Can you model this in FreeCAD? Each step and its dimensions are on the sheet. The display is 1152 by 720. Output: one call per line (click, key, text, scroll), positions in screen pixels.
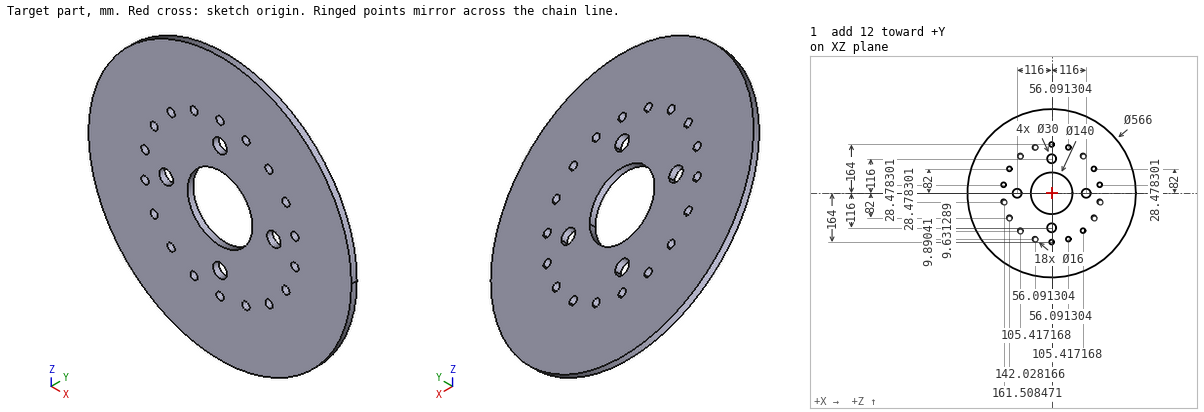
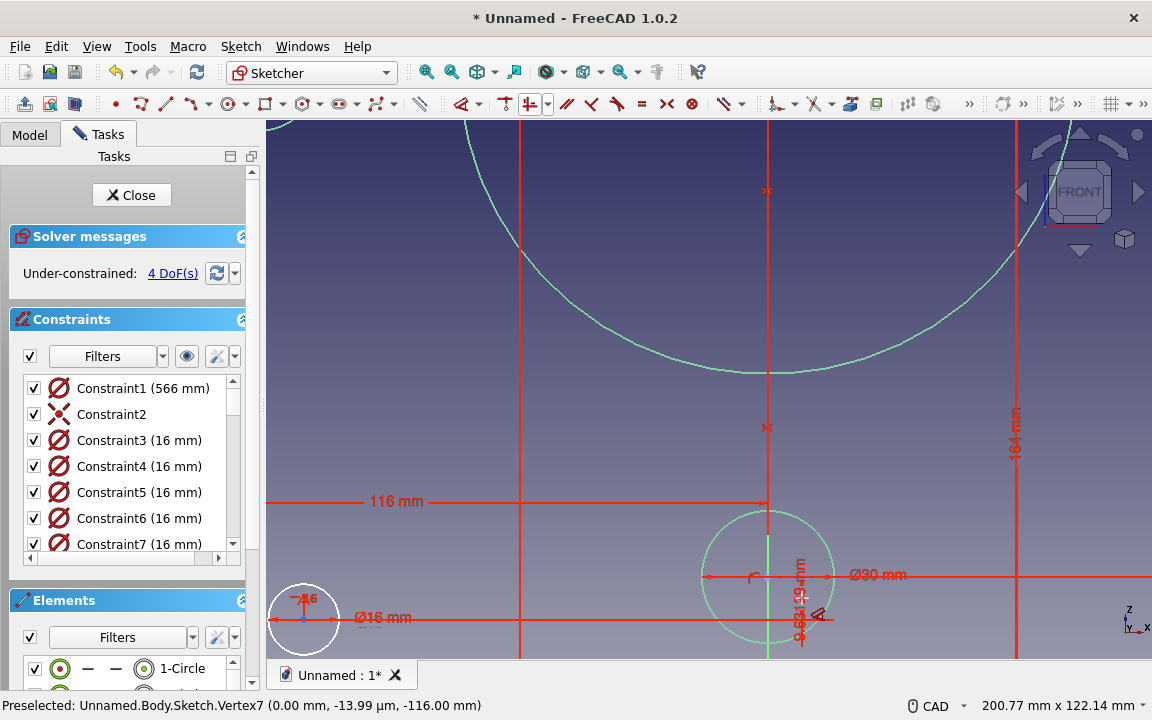
scroll(621, 440, down, 10)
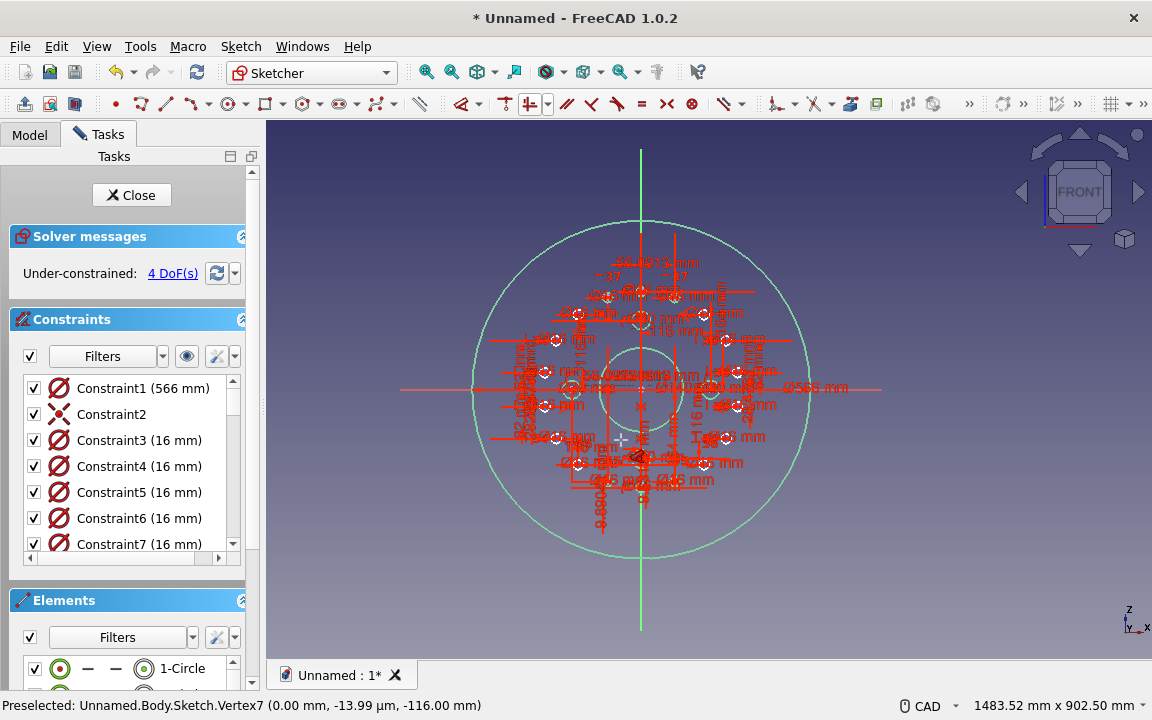
click(578, 465)
click(610, 523)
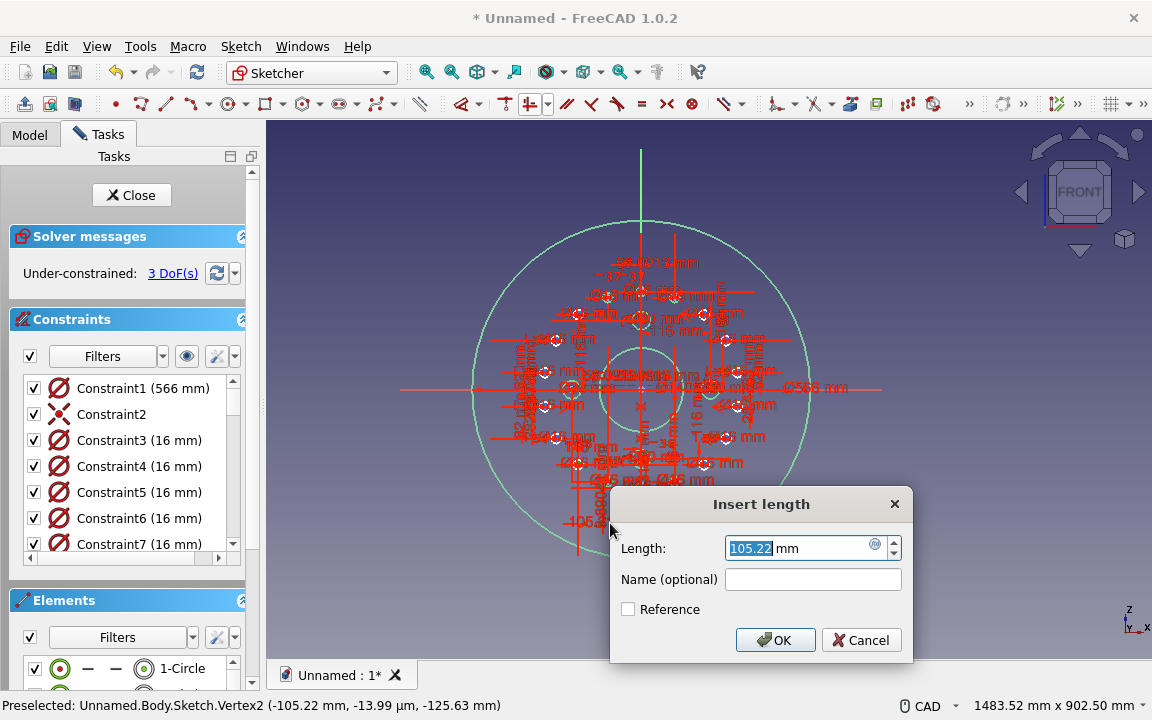
text(105.417168)
key(Return)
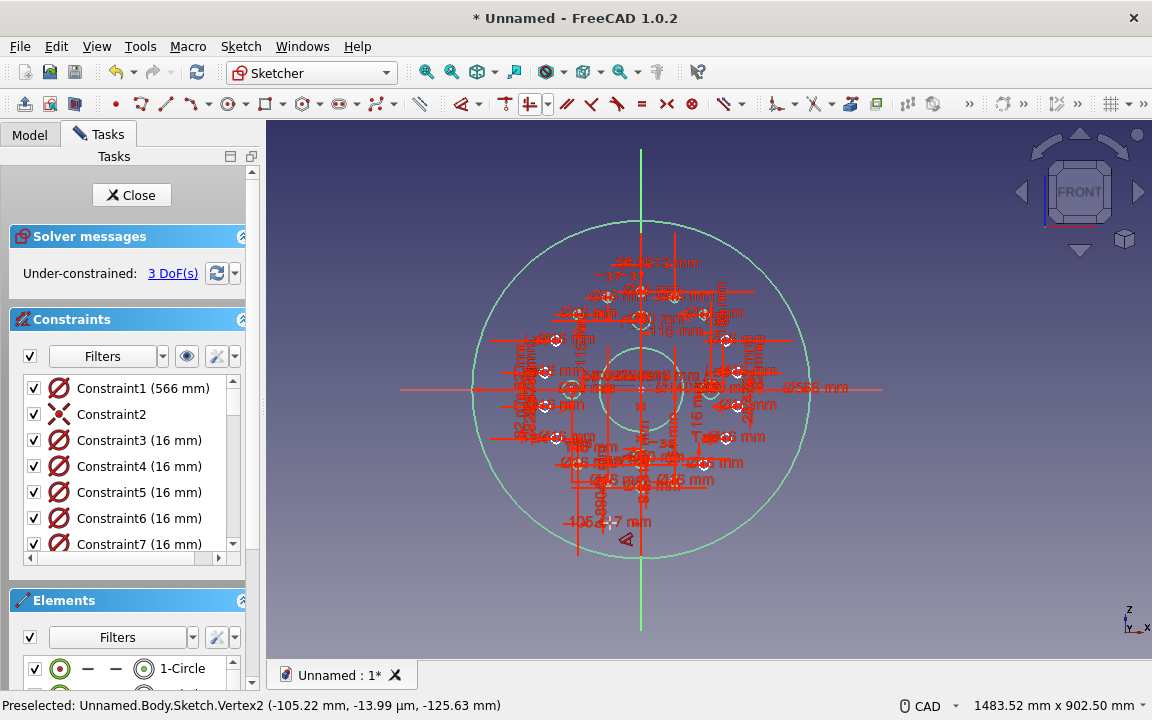
click(556, 439)
click(579, 284)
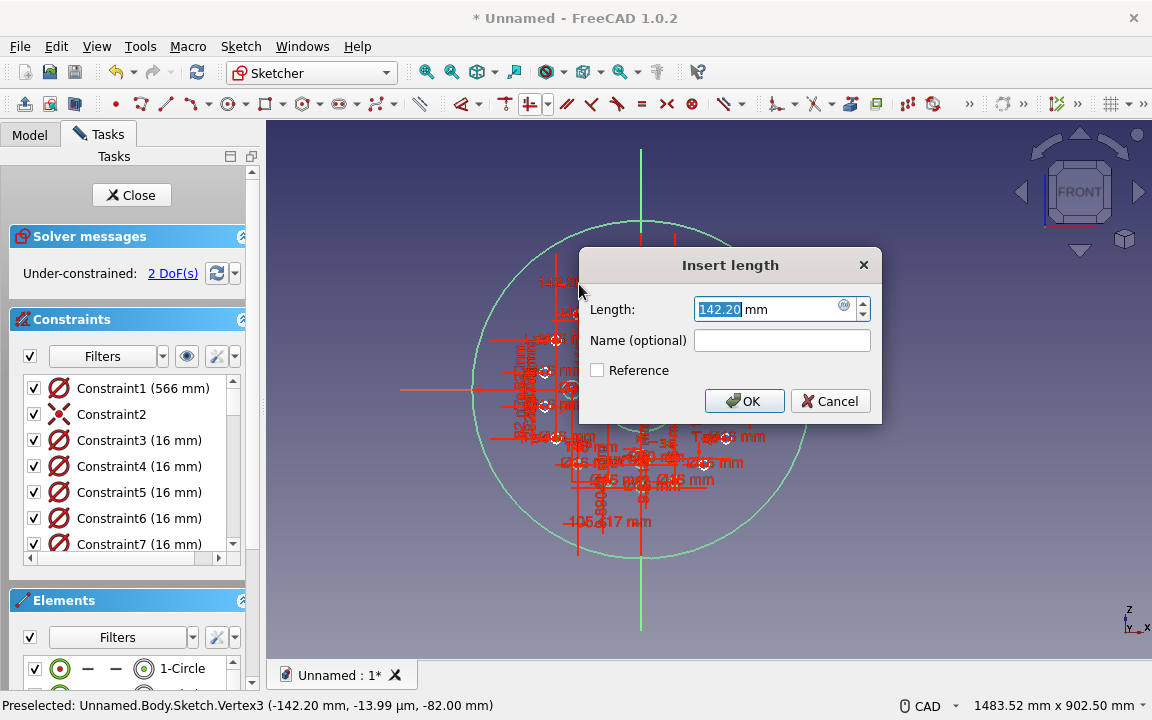
text(142.028166)
key(Return)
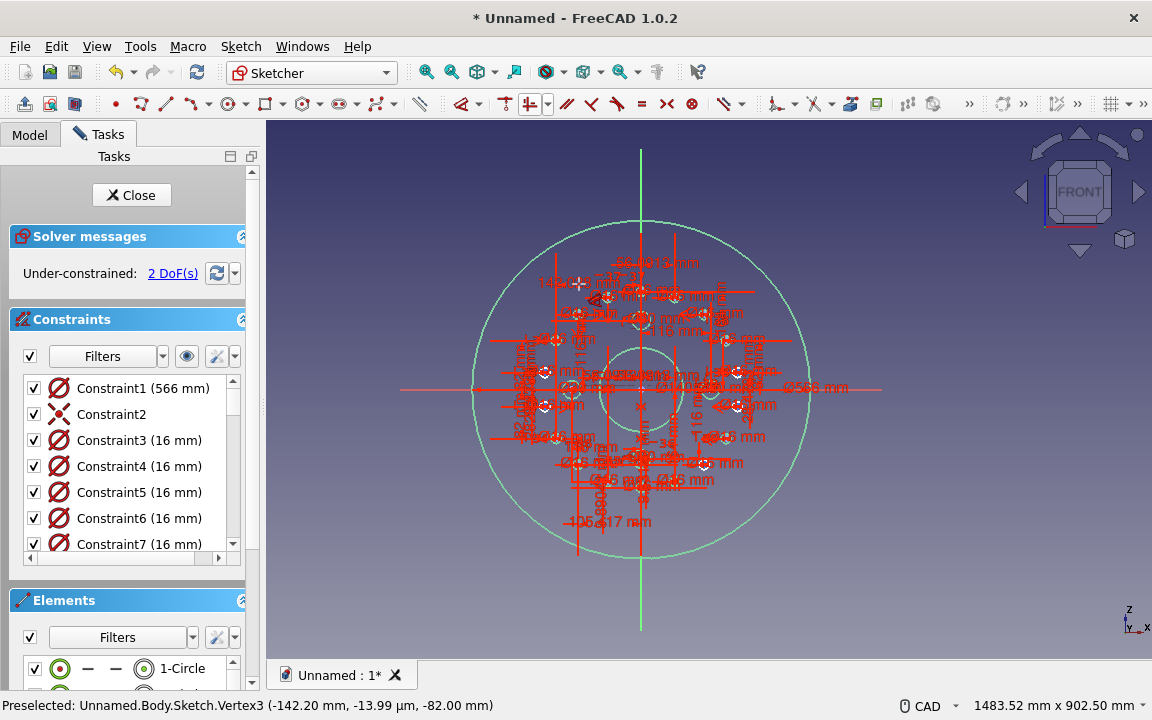
click(545, 407)
click(559, 308)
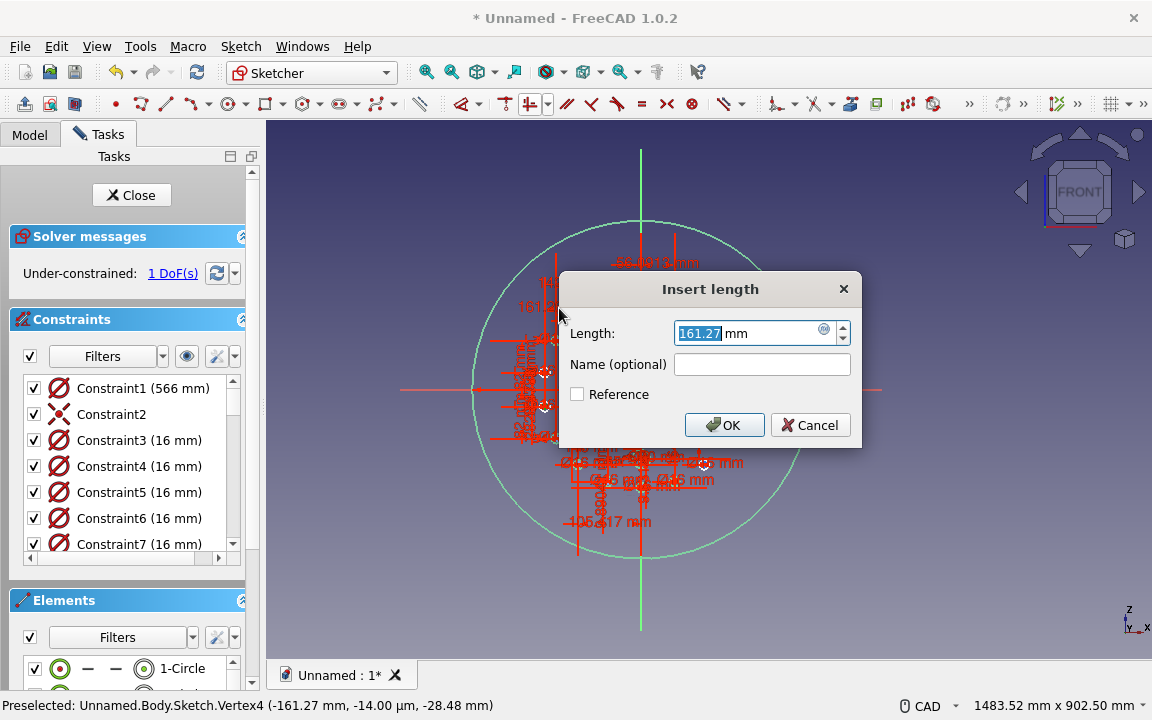
text(161.508471)
key(Return)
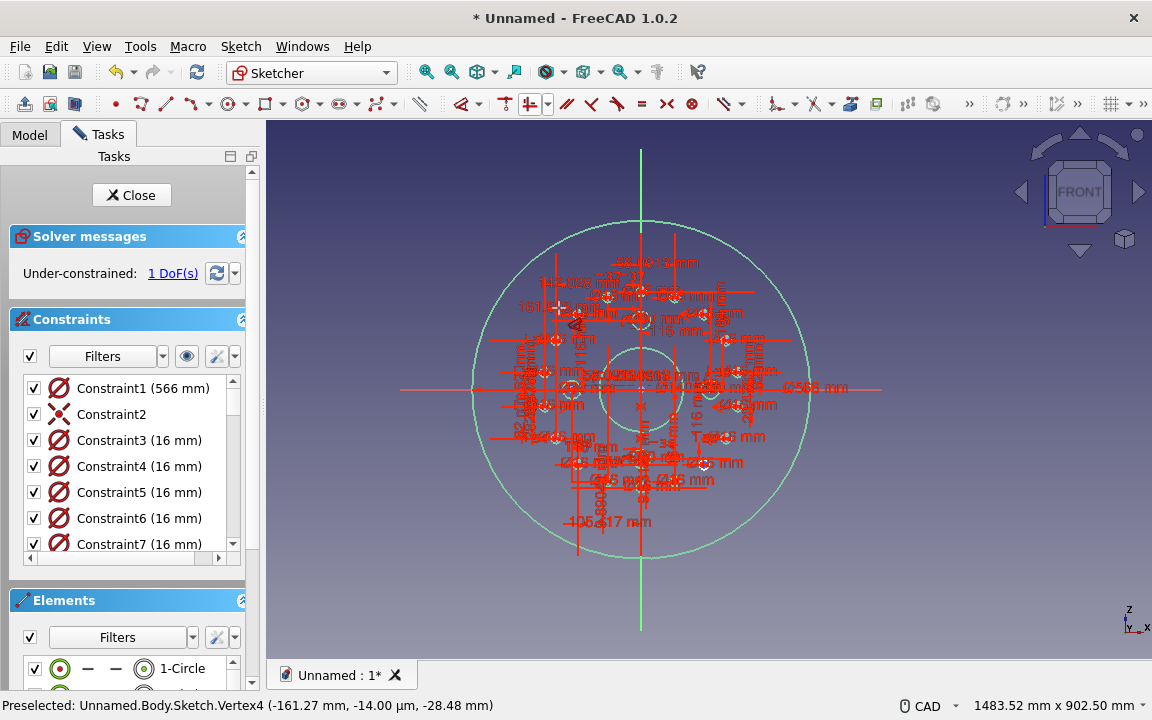
click(704, 465)
click(687, 499)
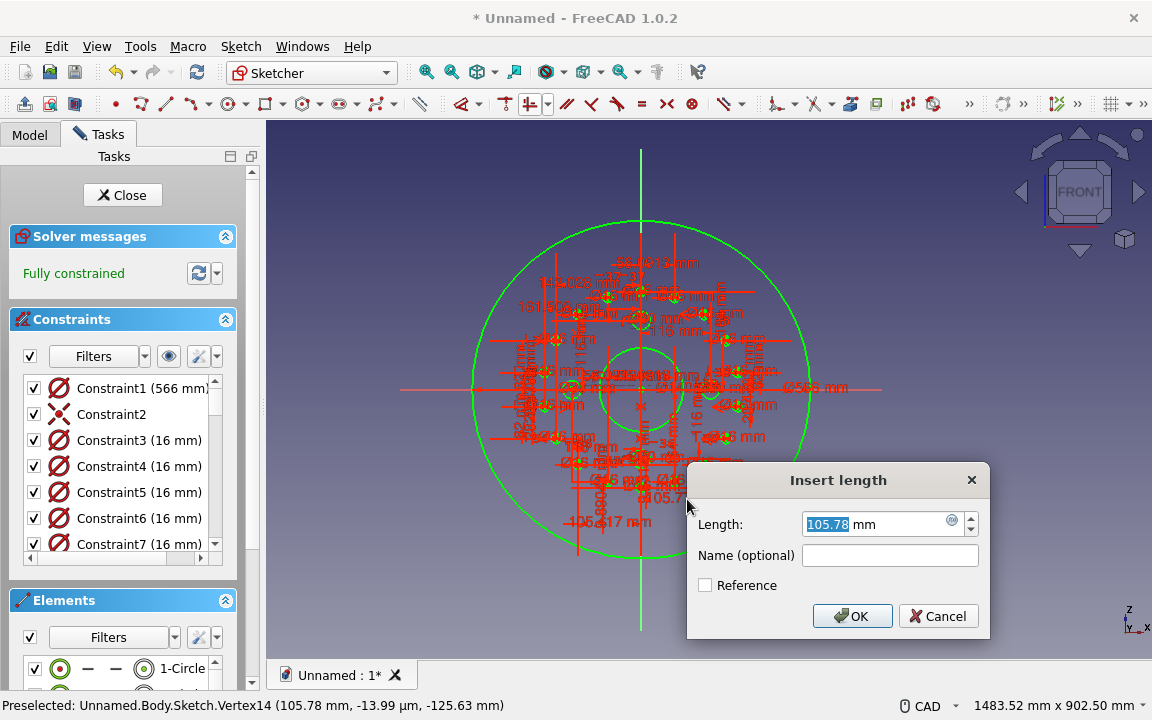
text(105.417168)
key(Return)
key(Escape)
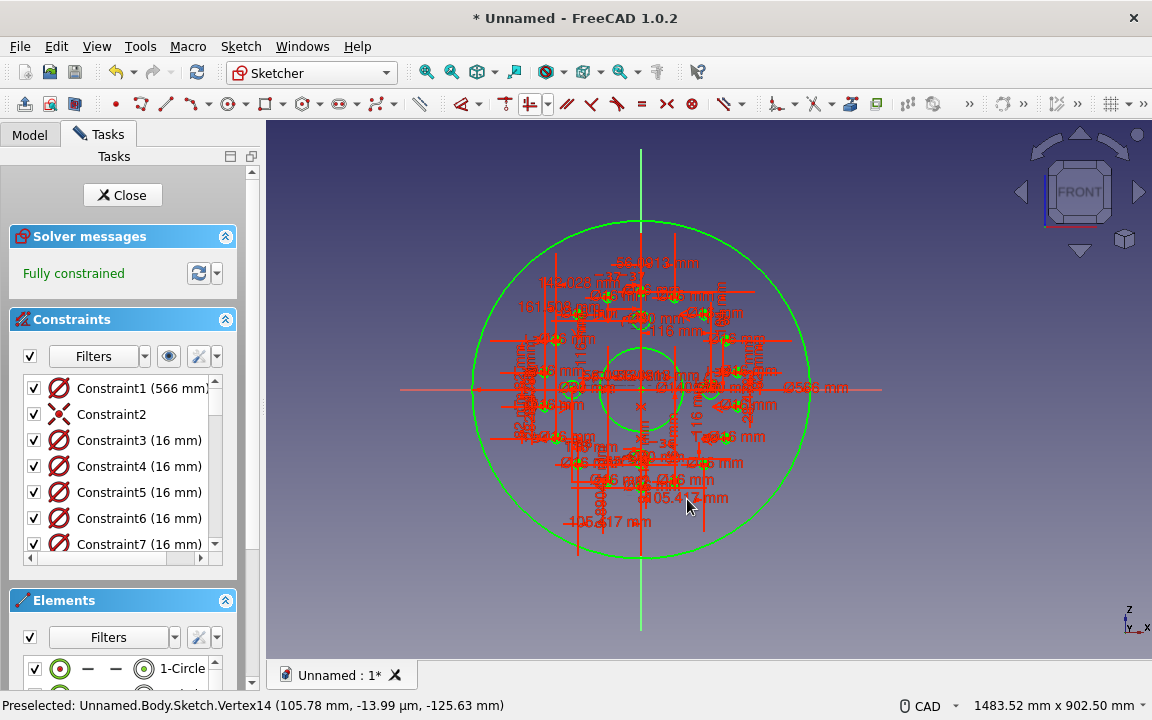
click(123, 195)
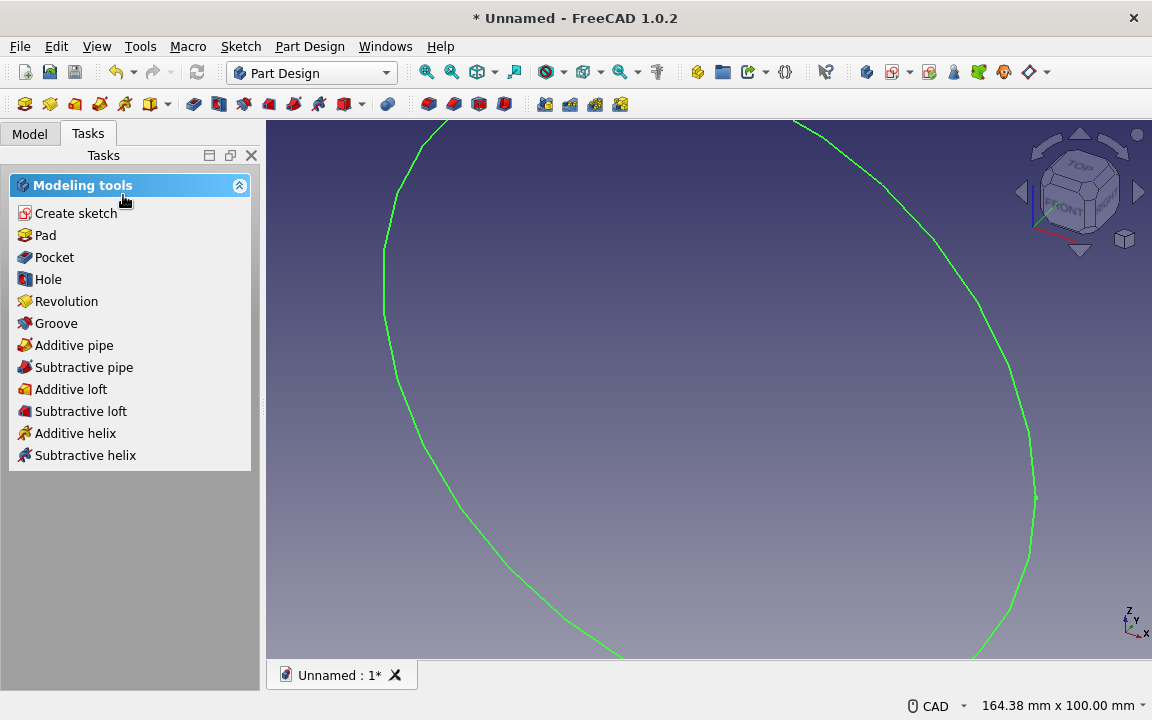
click(25, 104)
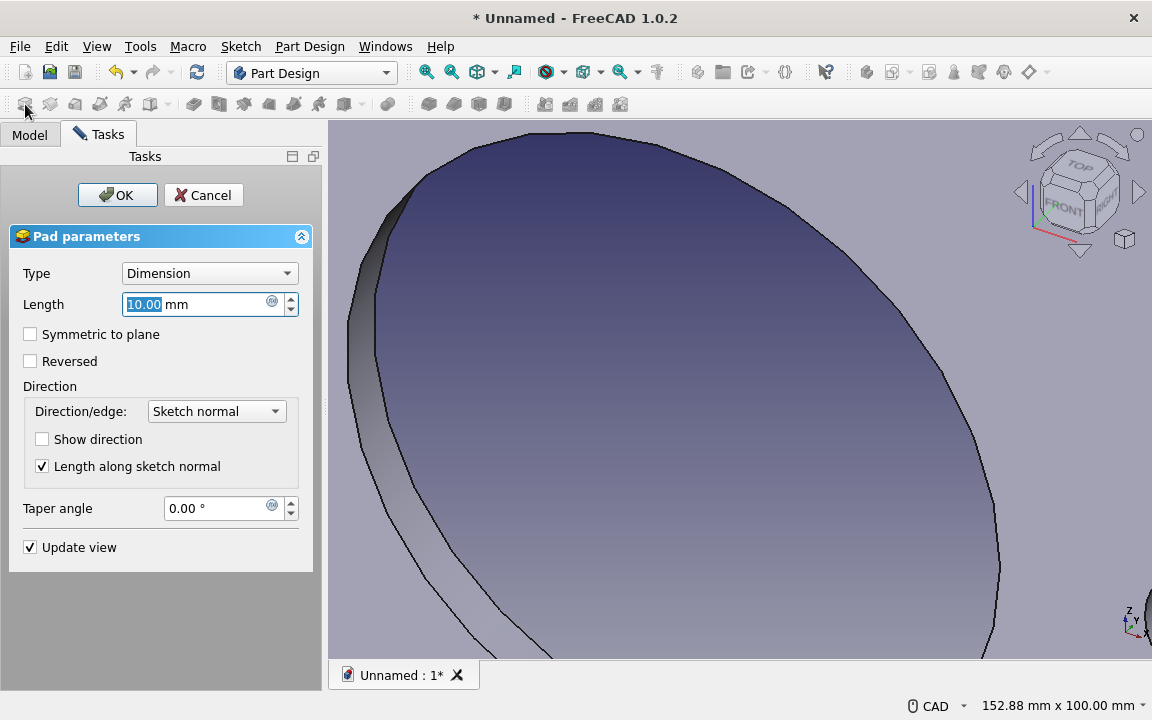
text(12)
key(Tab)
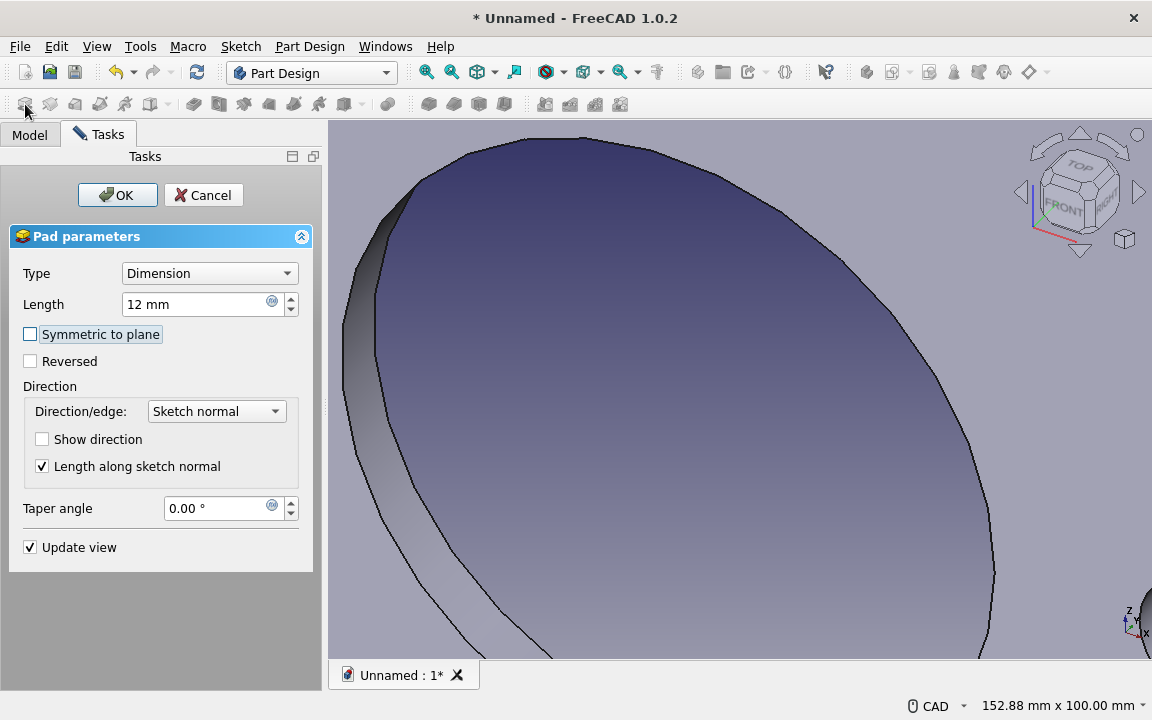
click(31, 361)